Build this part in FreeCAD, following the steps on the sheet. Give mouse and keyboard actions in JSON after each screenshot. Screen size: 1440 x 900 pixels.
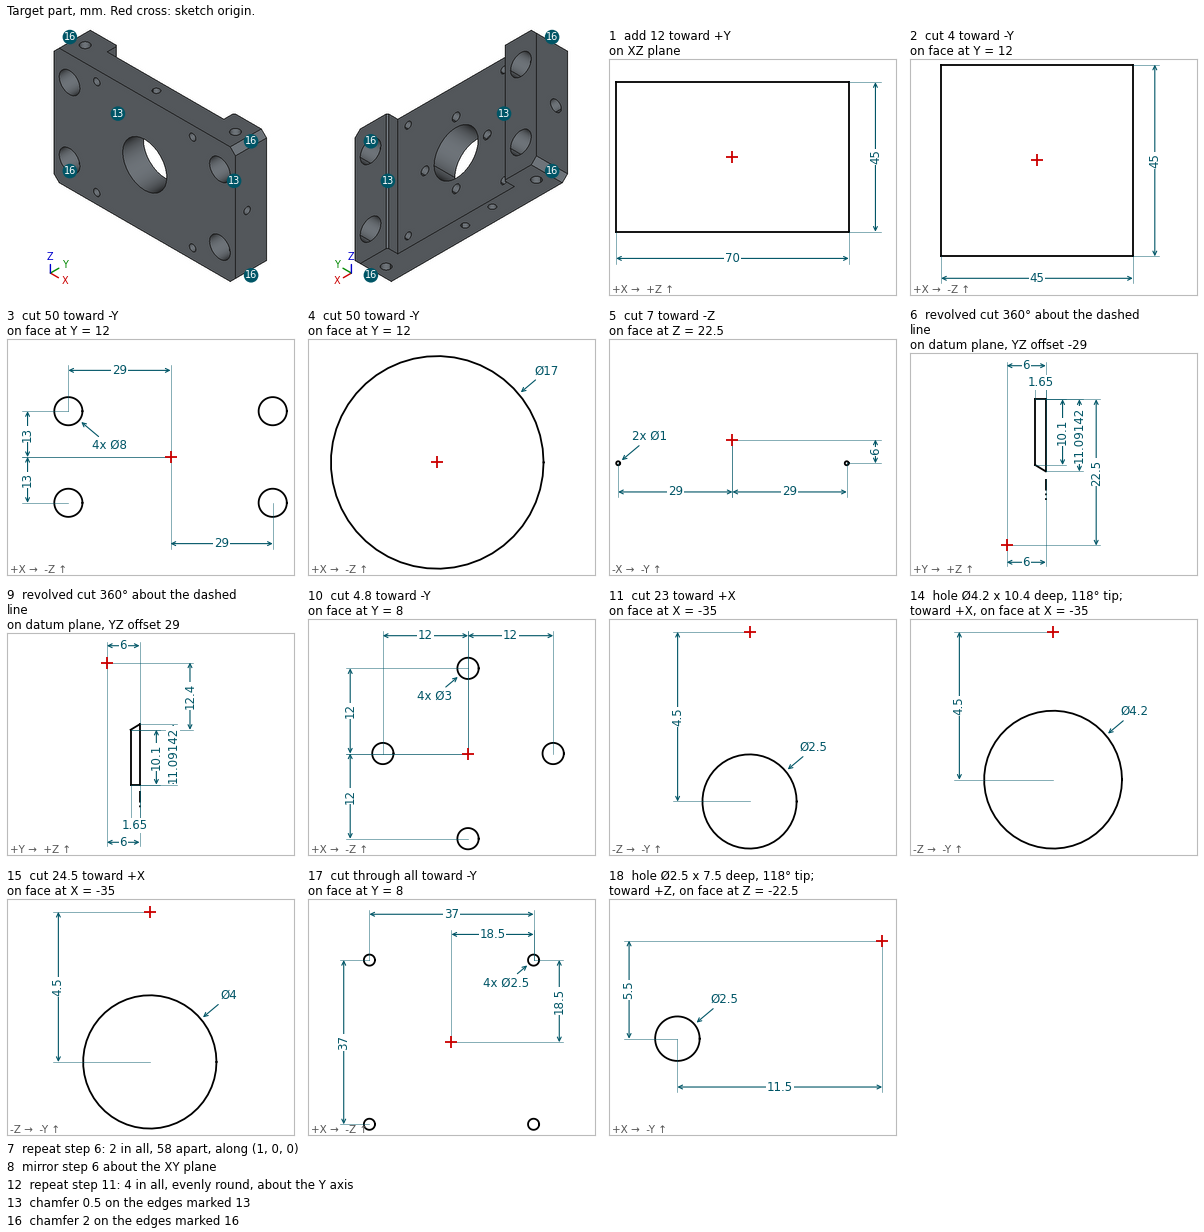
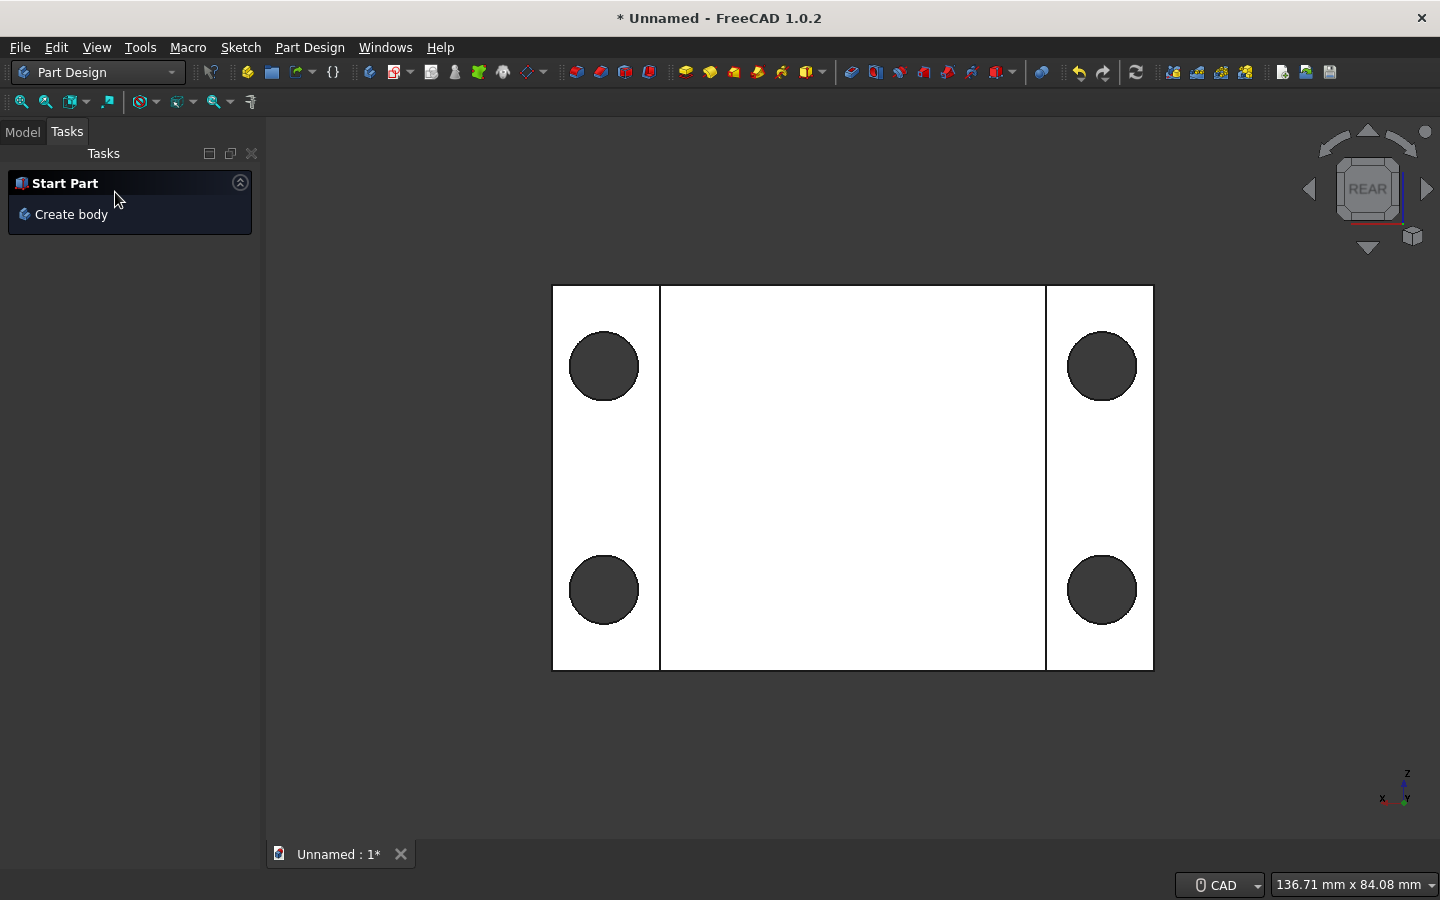
{"action": "left_click", "coordinate": [606, 477]}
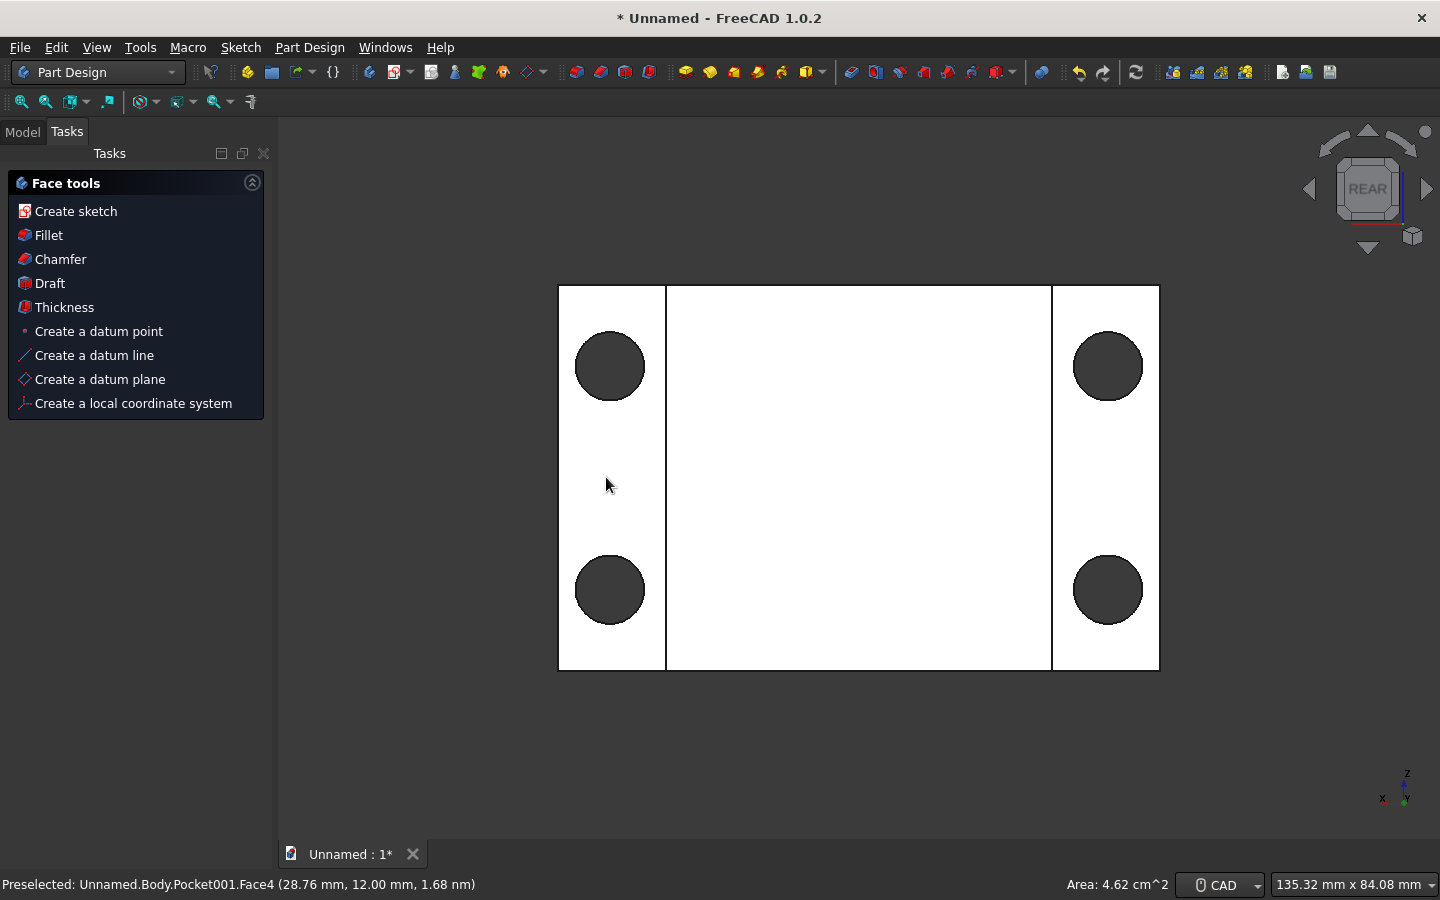
{"action": "left_click", "coordinate": [394, 72]}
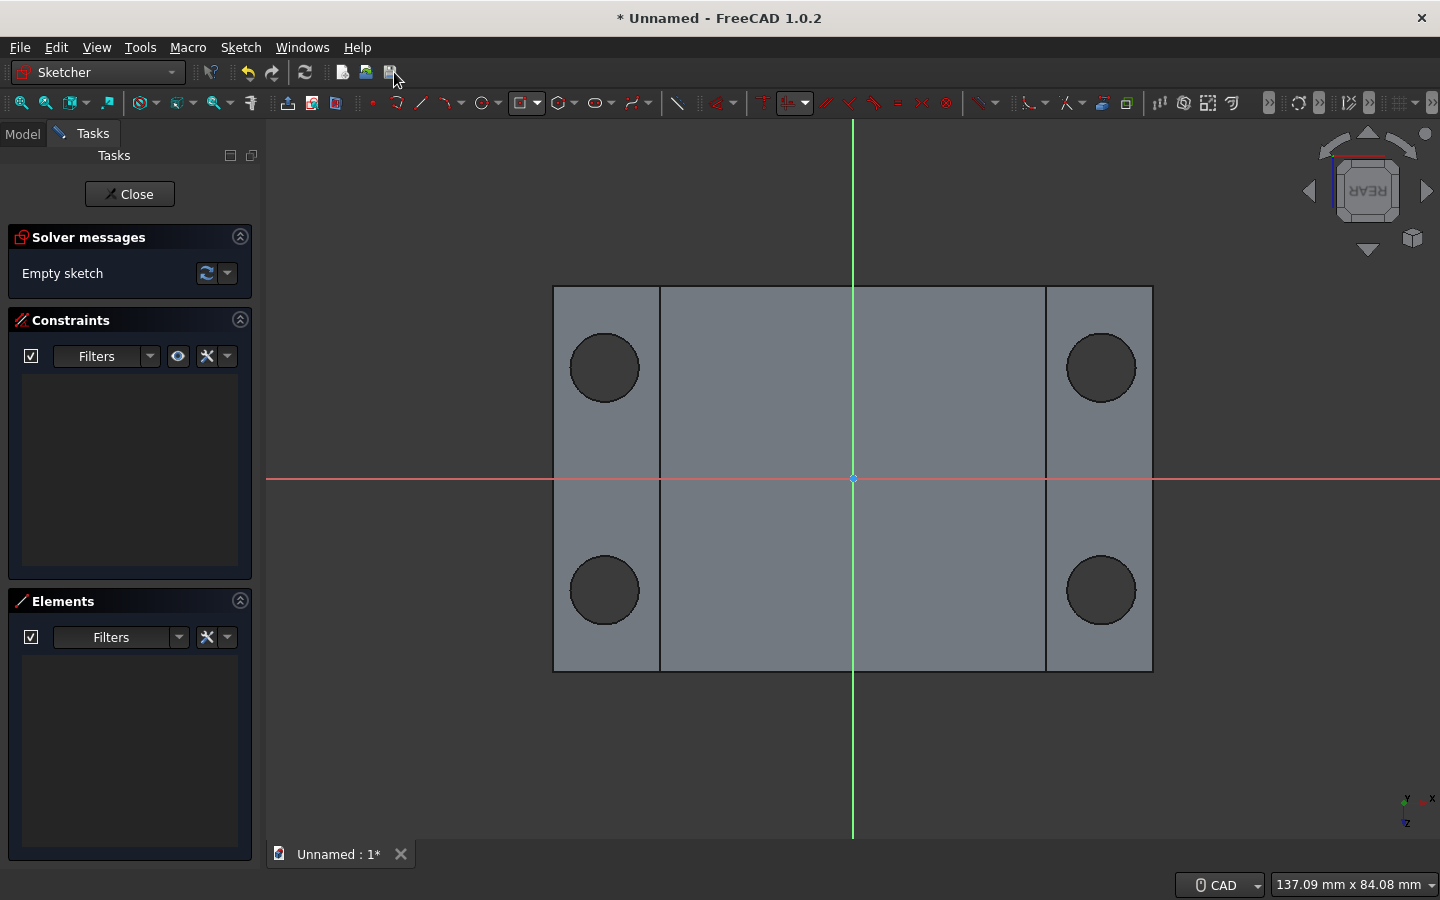
{"action": "scroll", "coordinate": [883, 479], "scroll_direction": "up", "scroll_amount": 6}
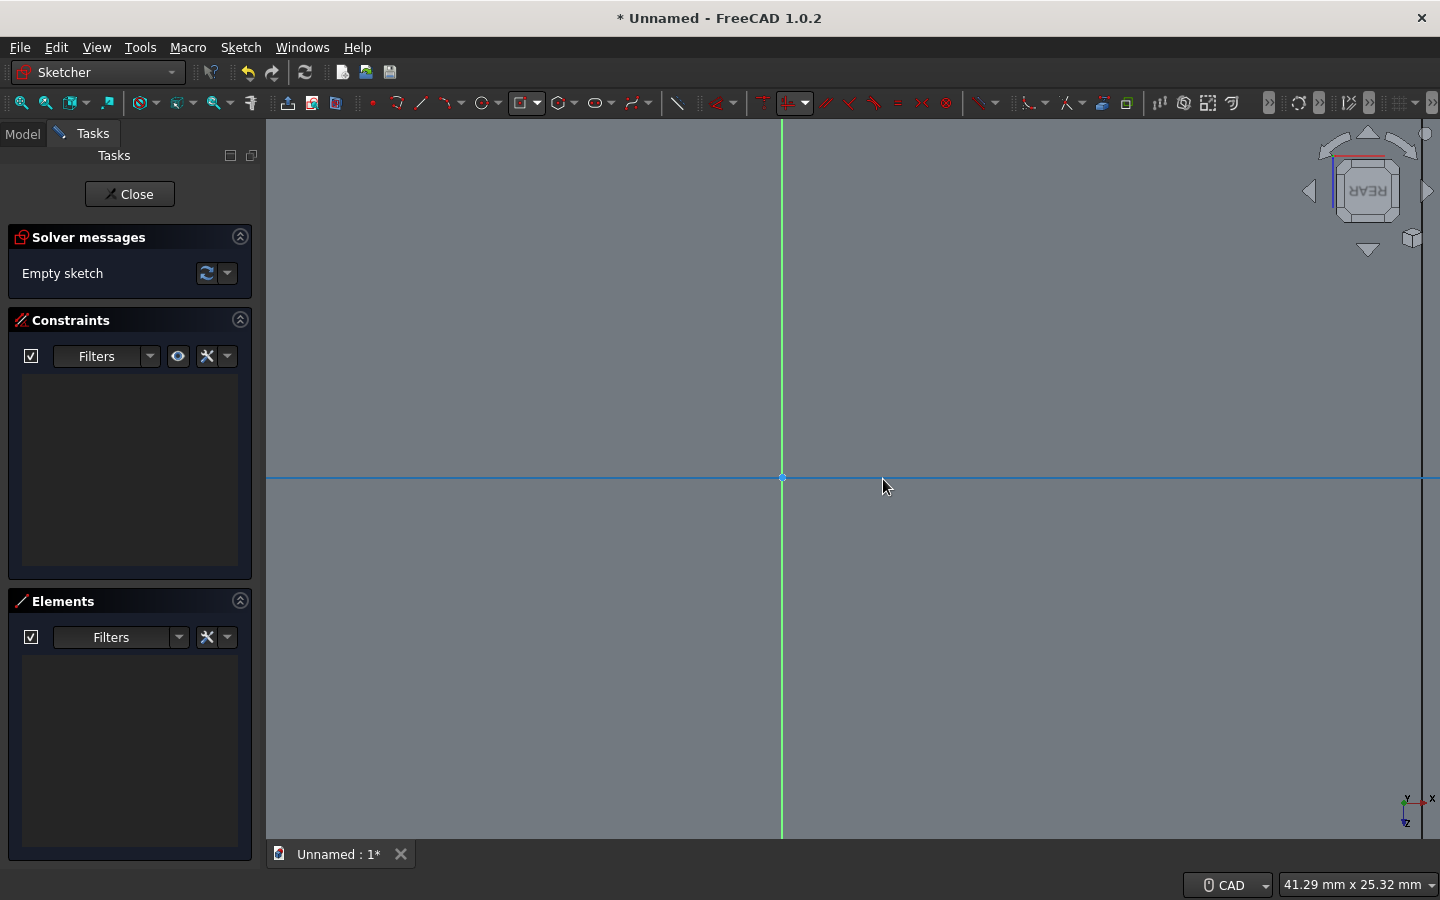
{"action": "left_click", "coordinate": [482, 104]}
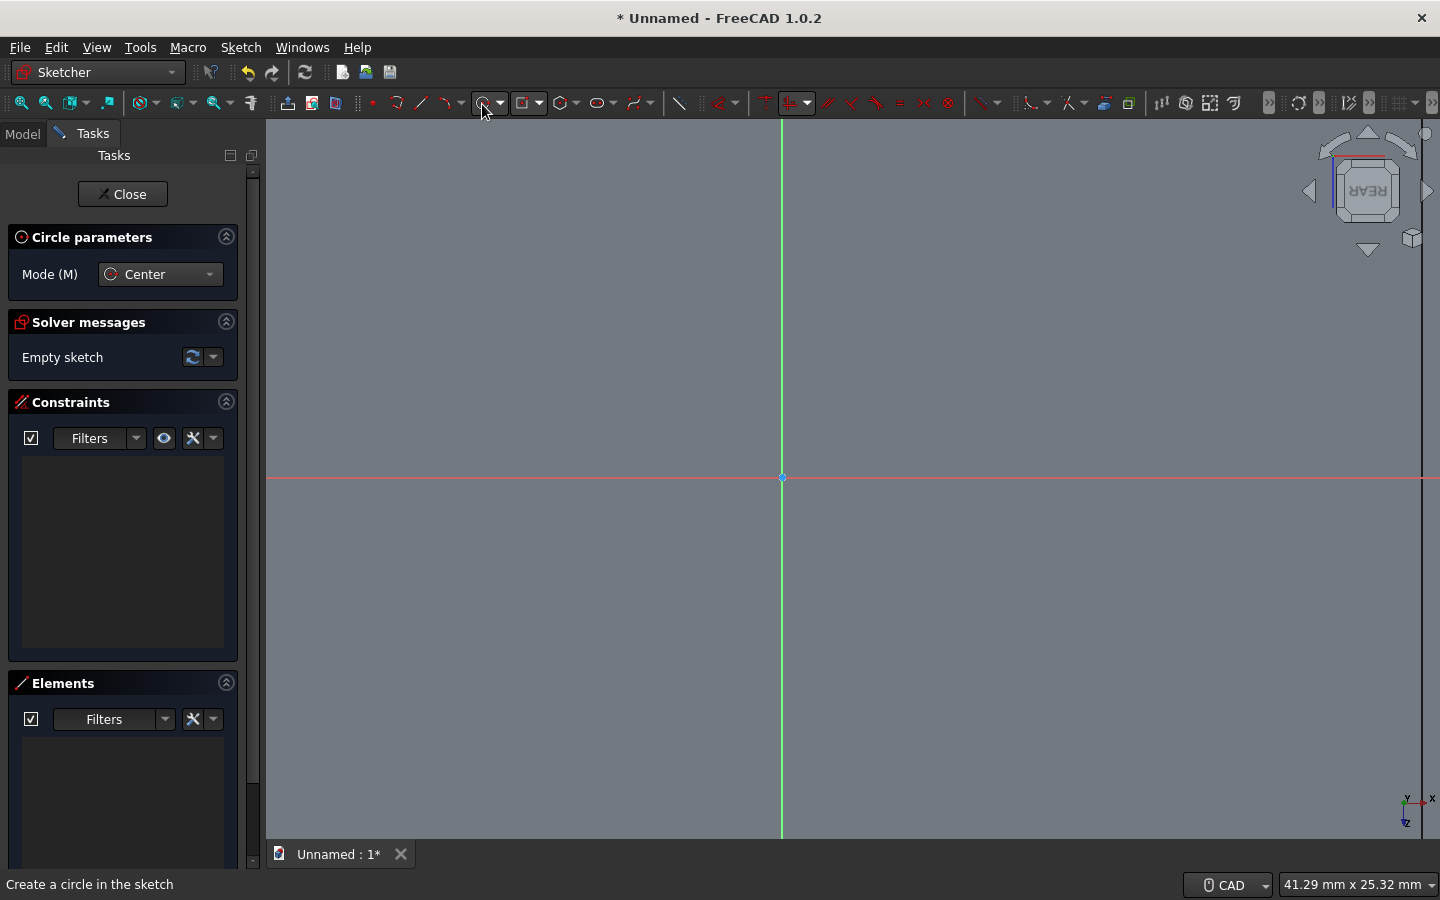
{"action": "left_click", "coordinate": [782, 478]}
{"action": "mouse_move", "coordinate": [953, 307]}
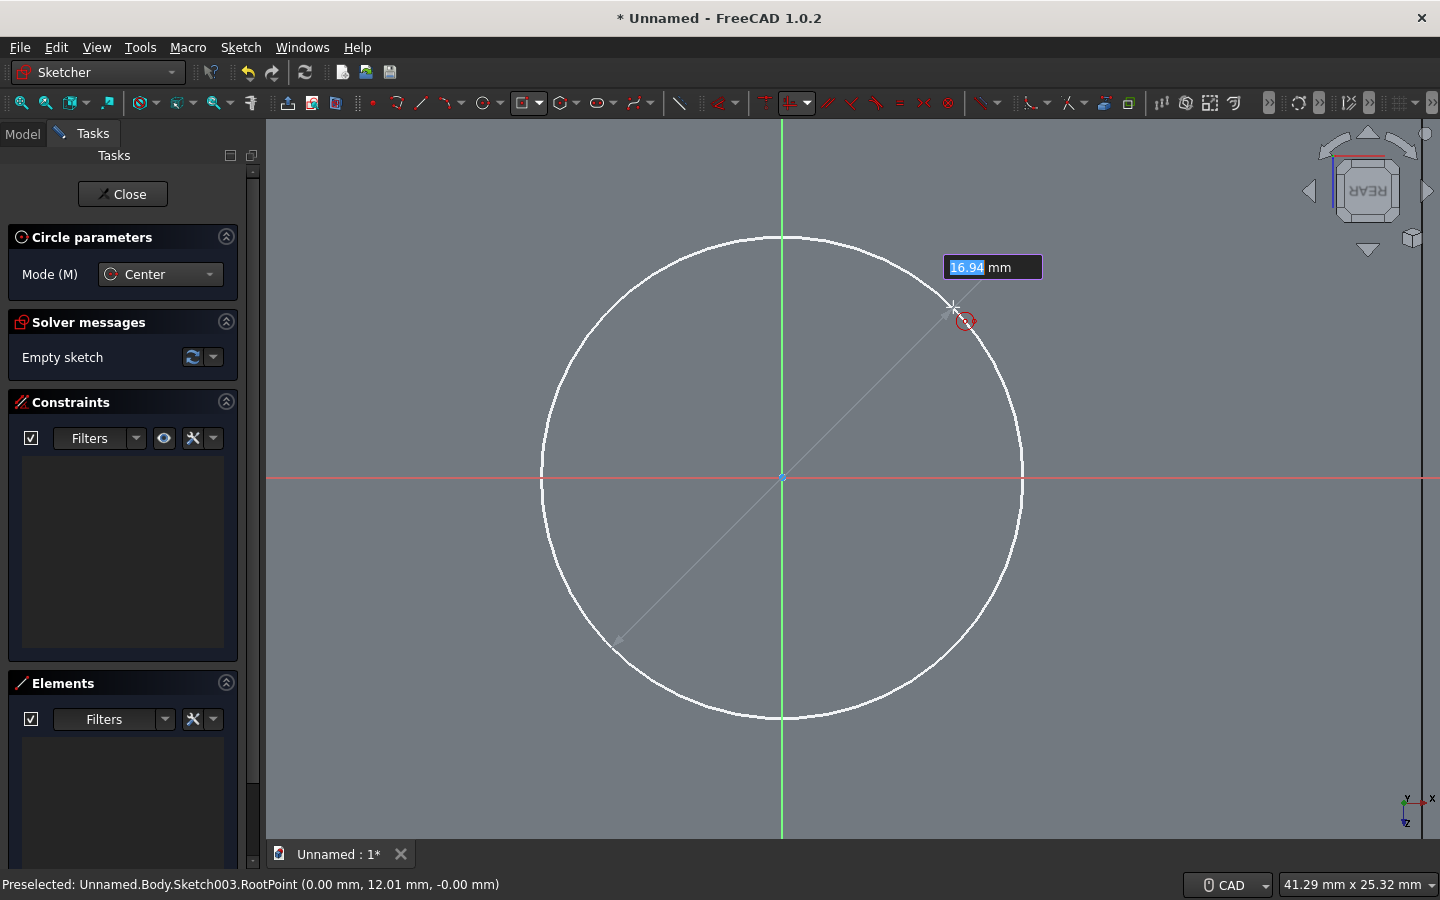
{"action": "type", "text": "17"}
{"action": "key", "text": "Return"}
{"action": "key", "text": "Escape"}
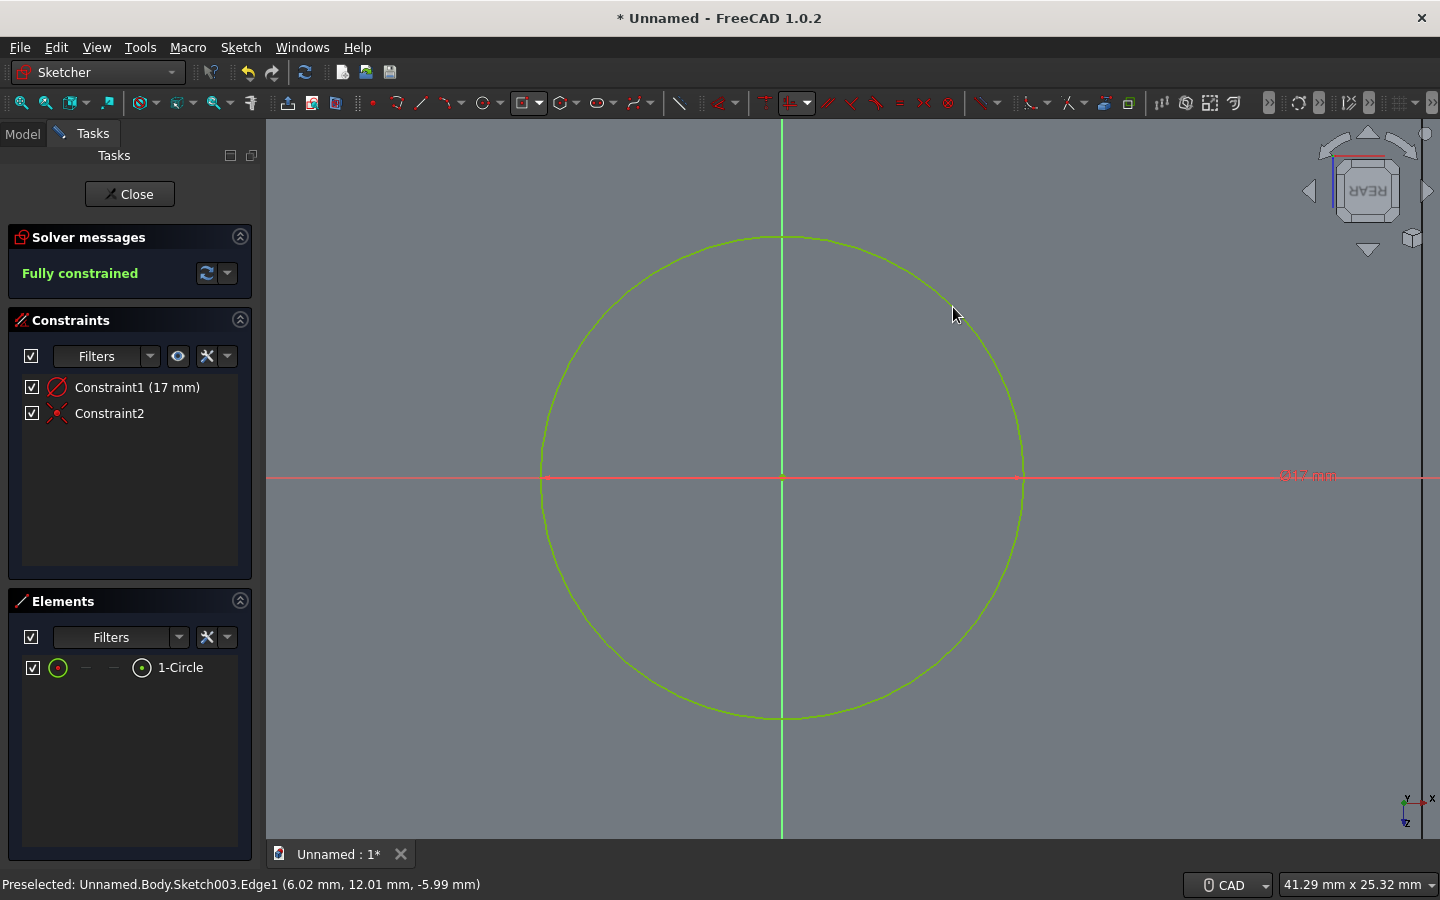
{"action": "left_click", "coordinate": [130, 194]}